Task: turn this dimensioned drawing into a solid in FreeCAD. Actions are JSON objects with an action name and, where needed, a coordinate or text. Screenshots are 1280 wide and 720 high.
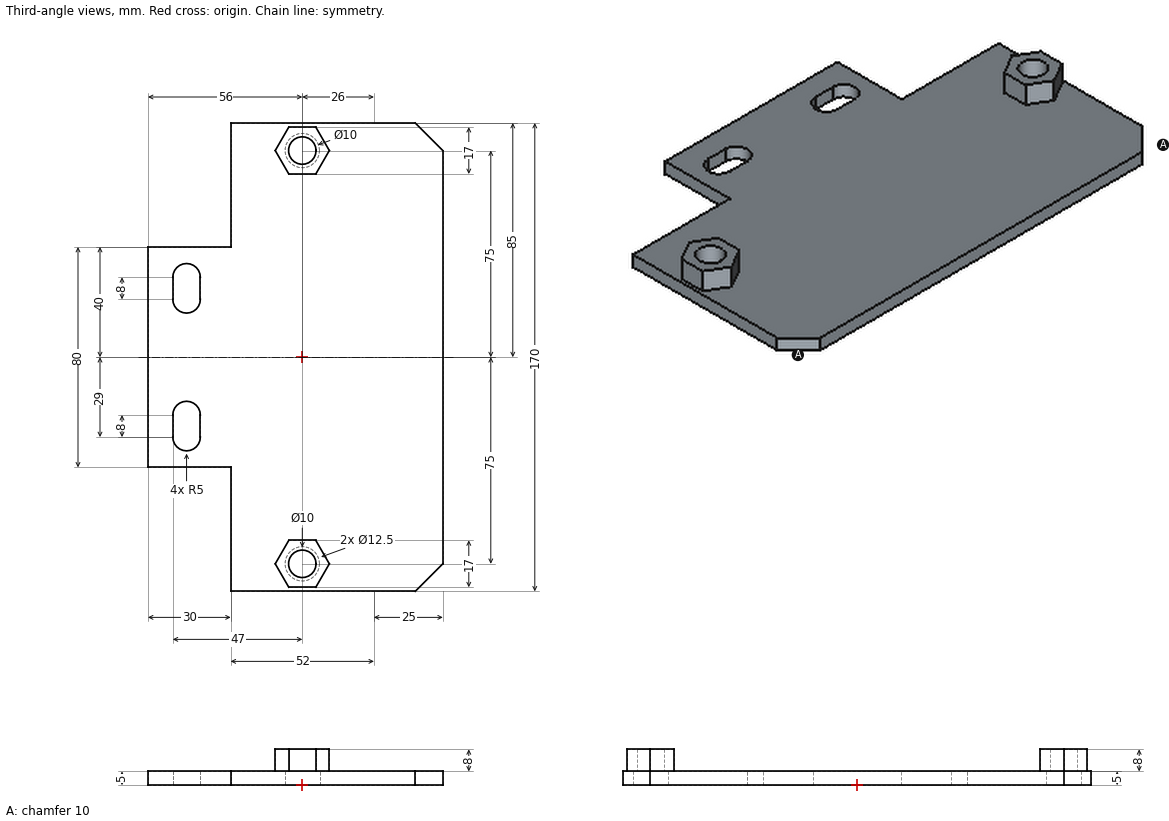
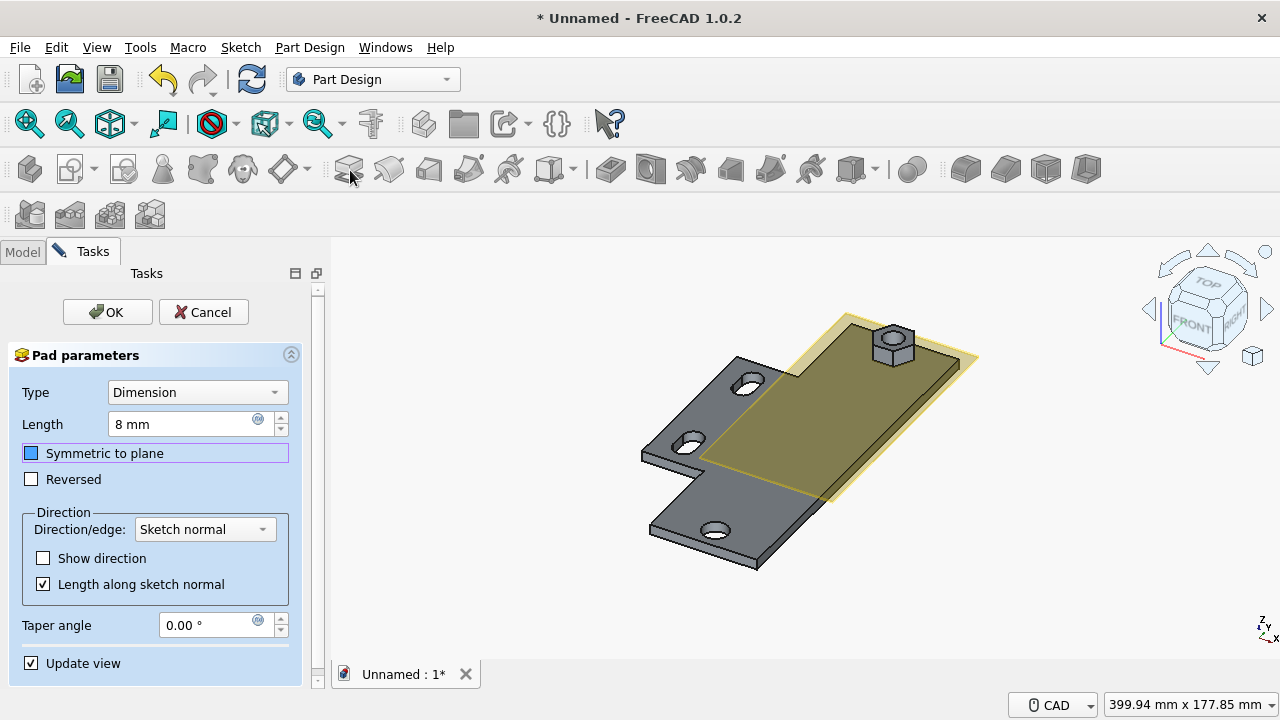
{"action": "left_click", "coordinate": [108, 312]}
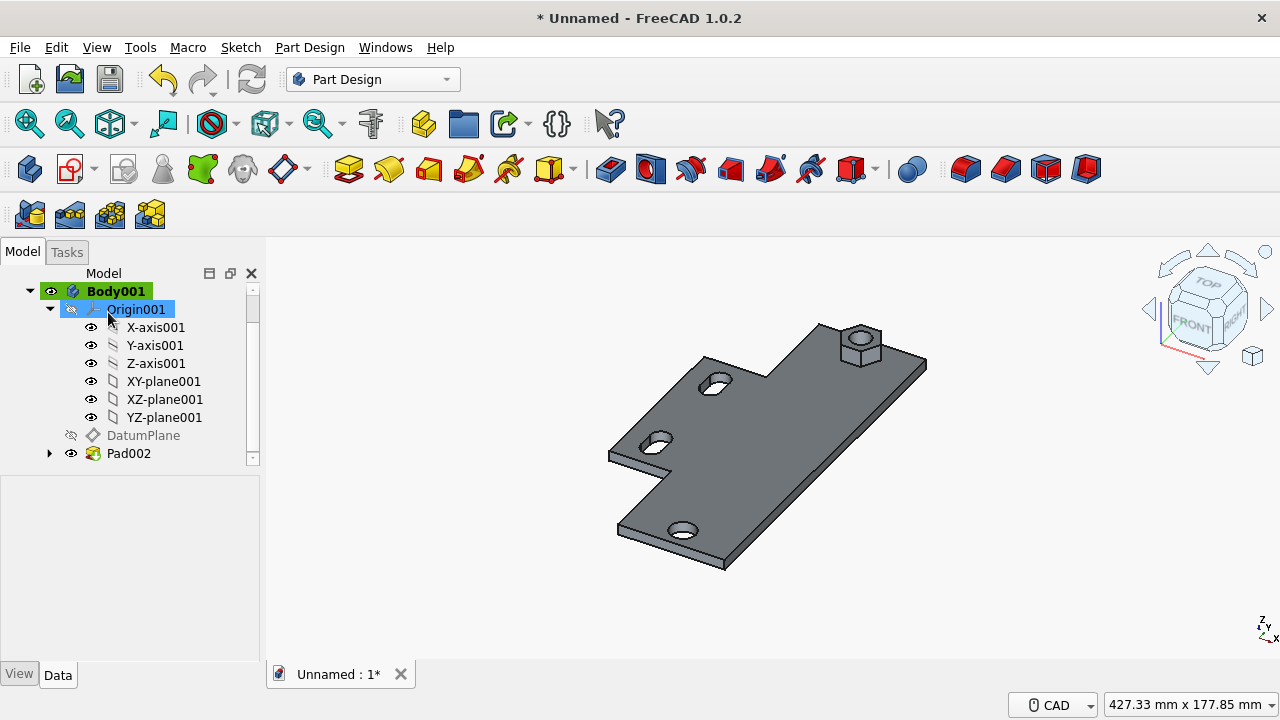
{"action": "left_click", "coordinate": [30, 124]}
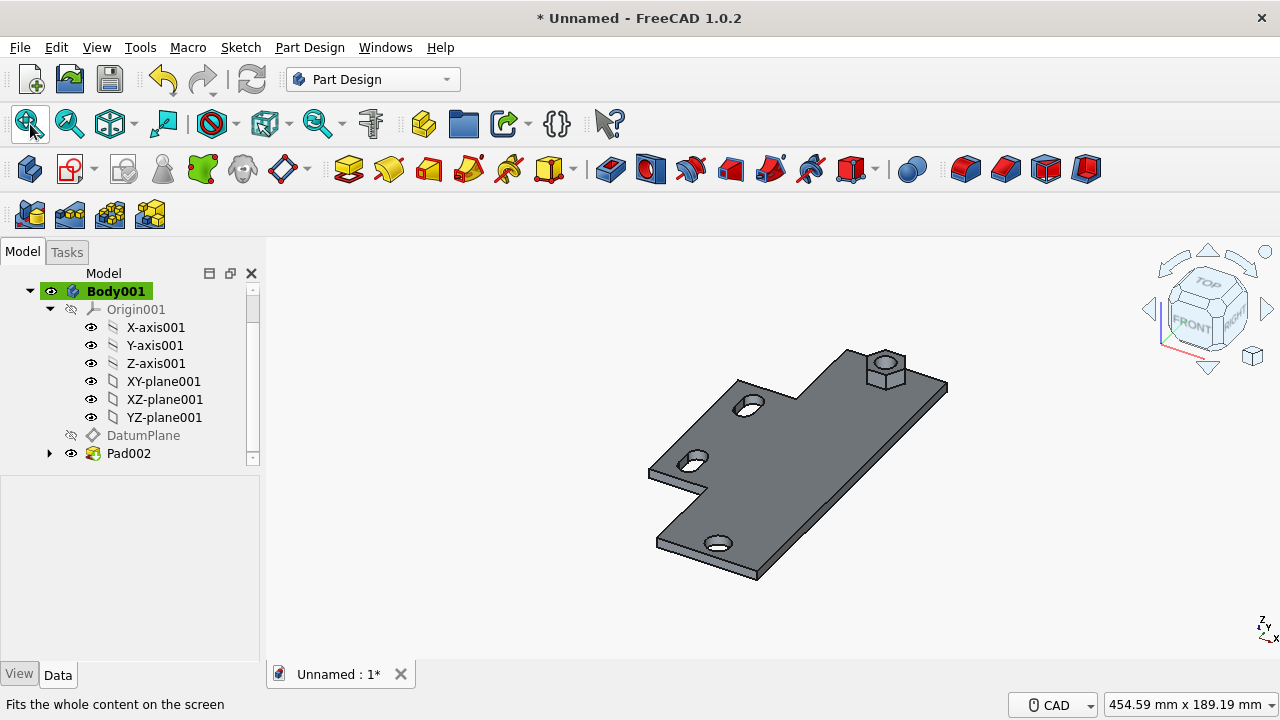
{"action": "left_click", "coordinate": [30, 170]}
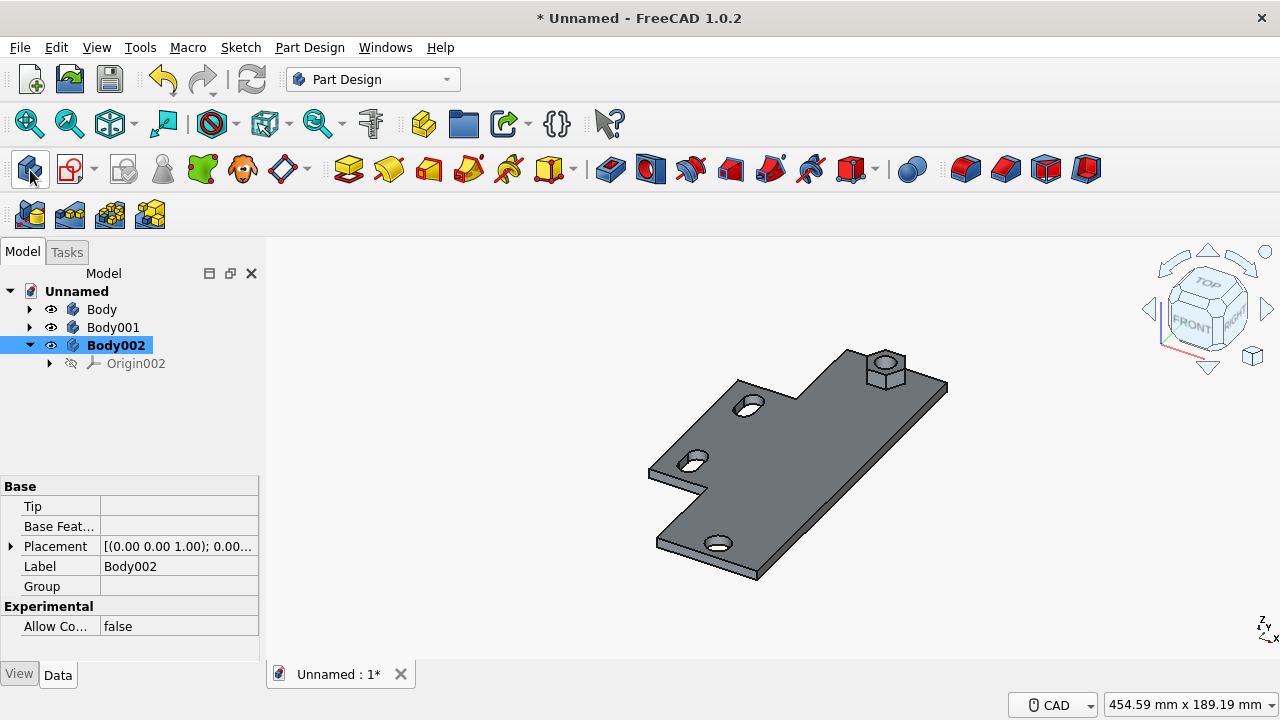
{"action": "left_click", "coordinate": [50, 363]}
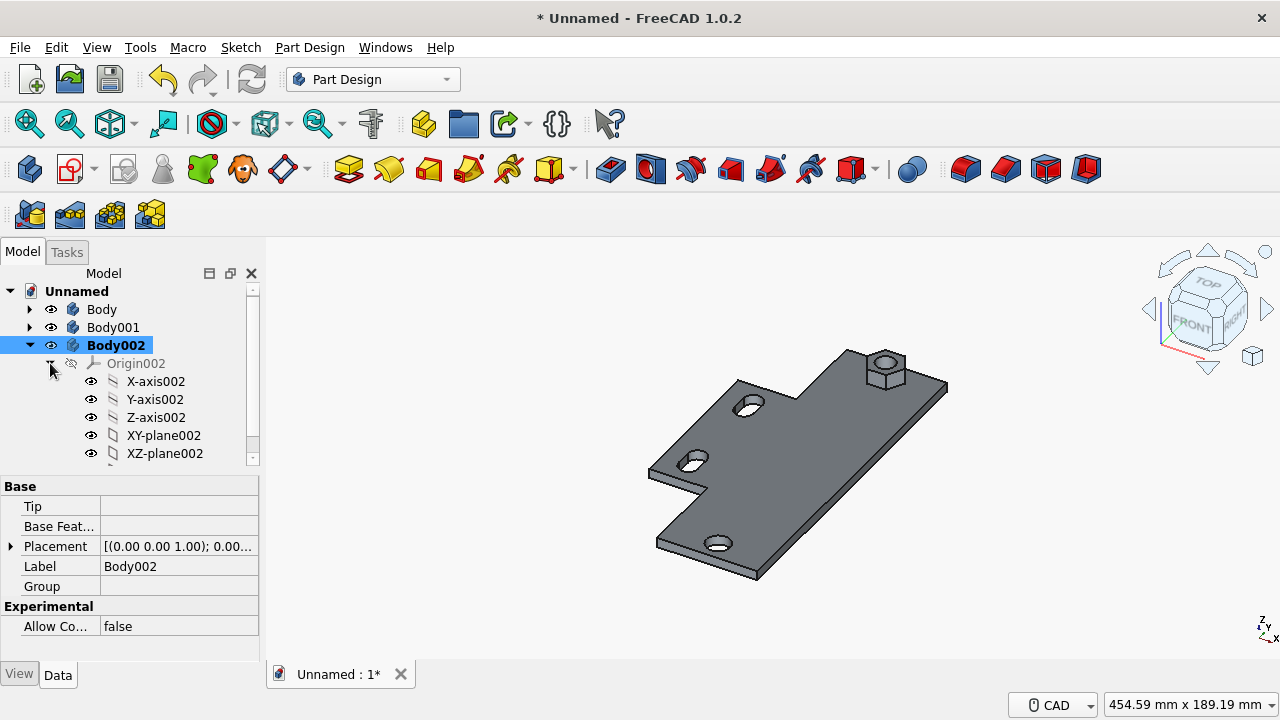
{"action": "left_click", "coordinate": [136, 435]}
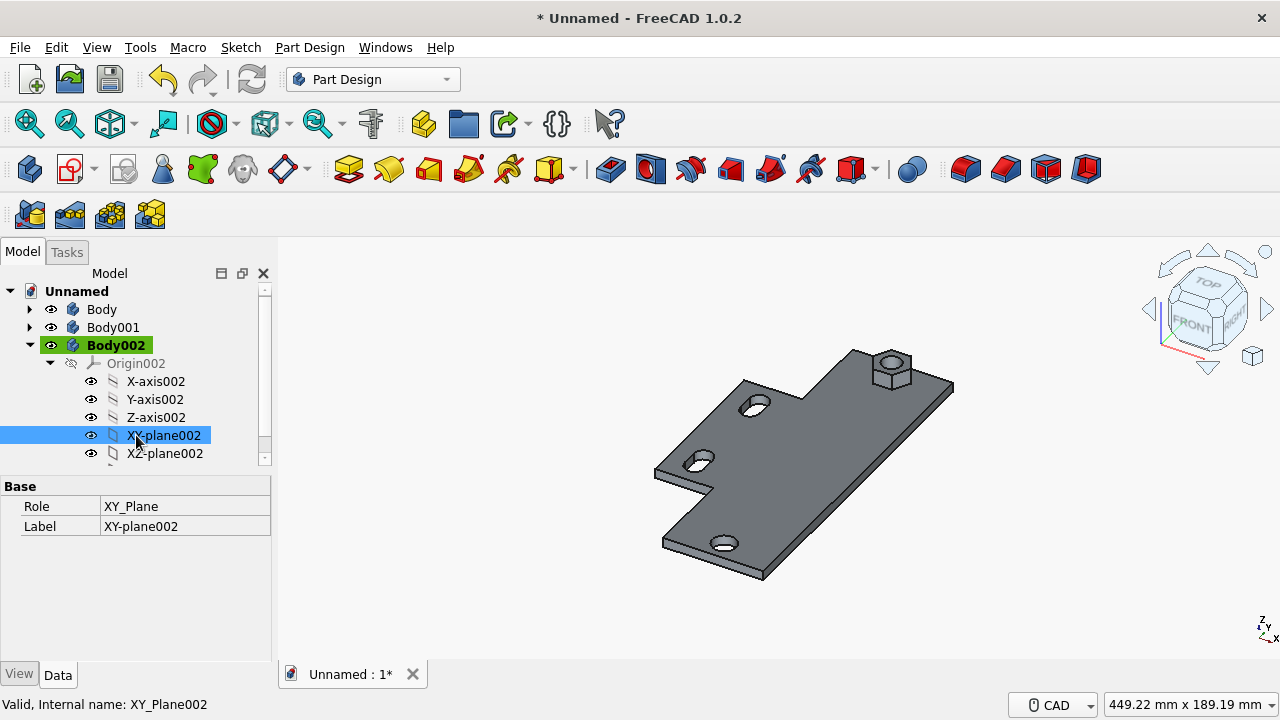
{"action": "left_click", "coordinate": [284, 170]}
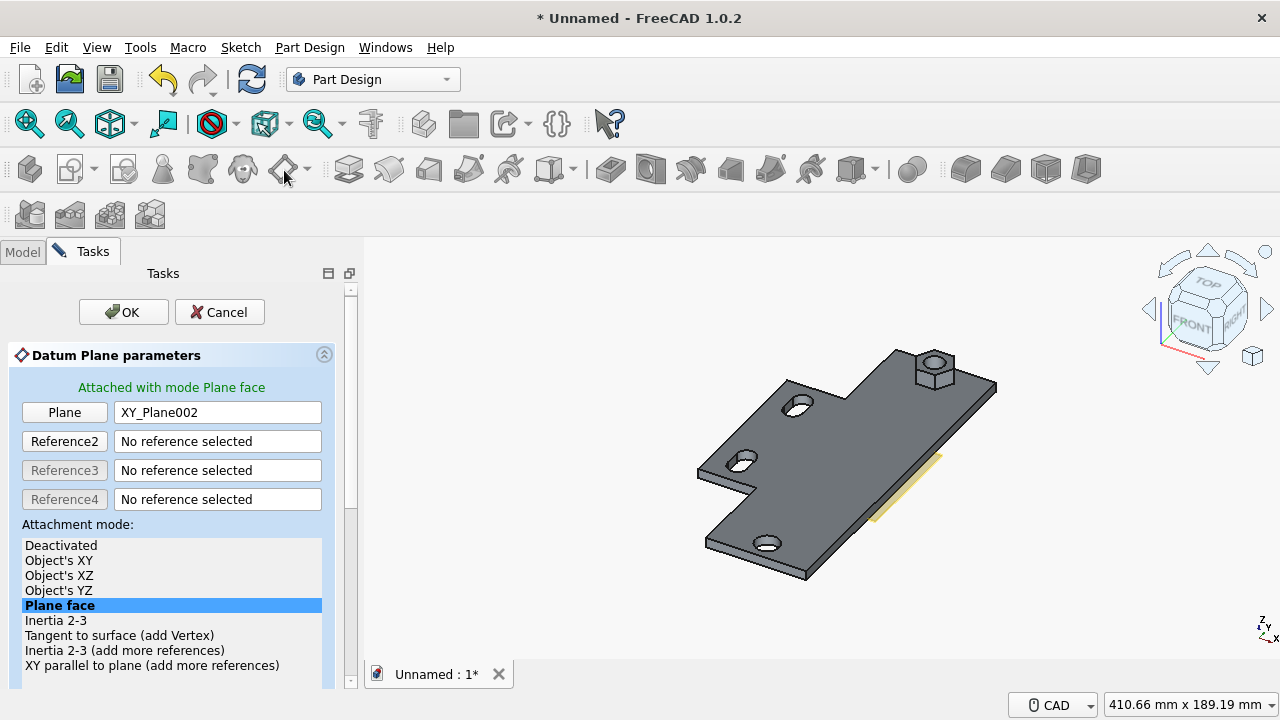
{"action": "scroll", "coordinate": [351, 486], "scroll_direction": "down", "scroll_amount": 4}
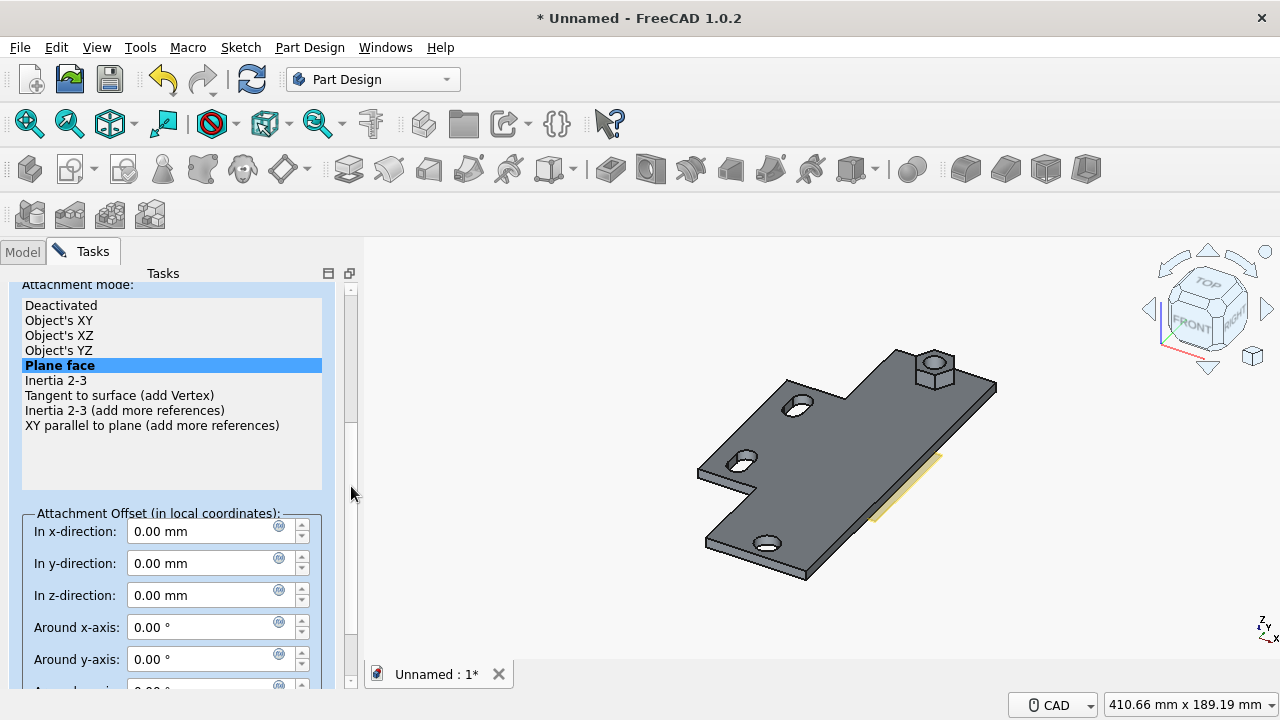
{"action": "triple_click", "coordinate": [210, 595]}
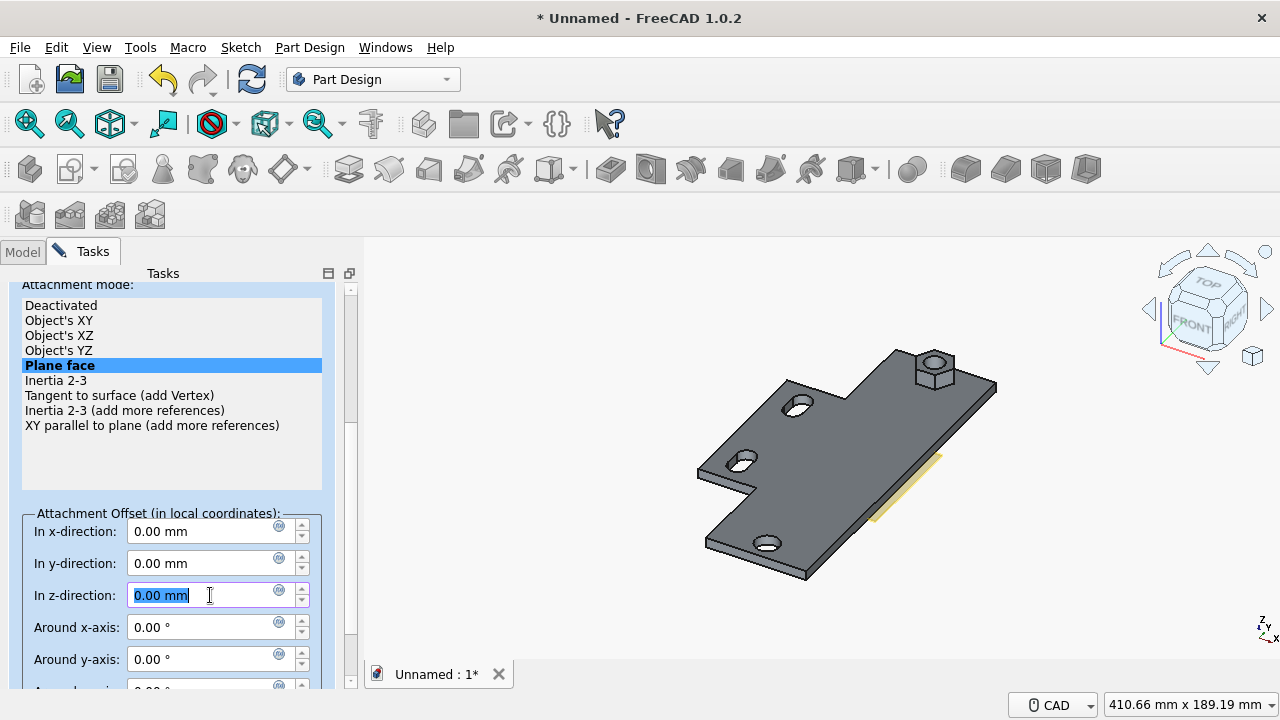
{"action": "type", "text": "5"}
{"action": "key", "text": "Tab"}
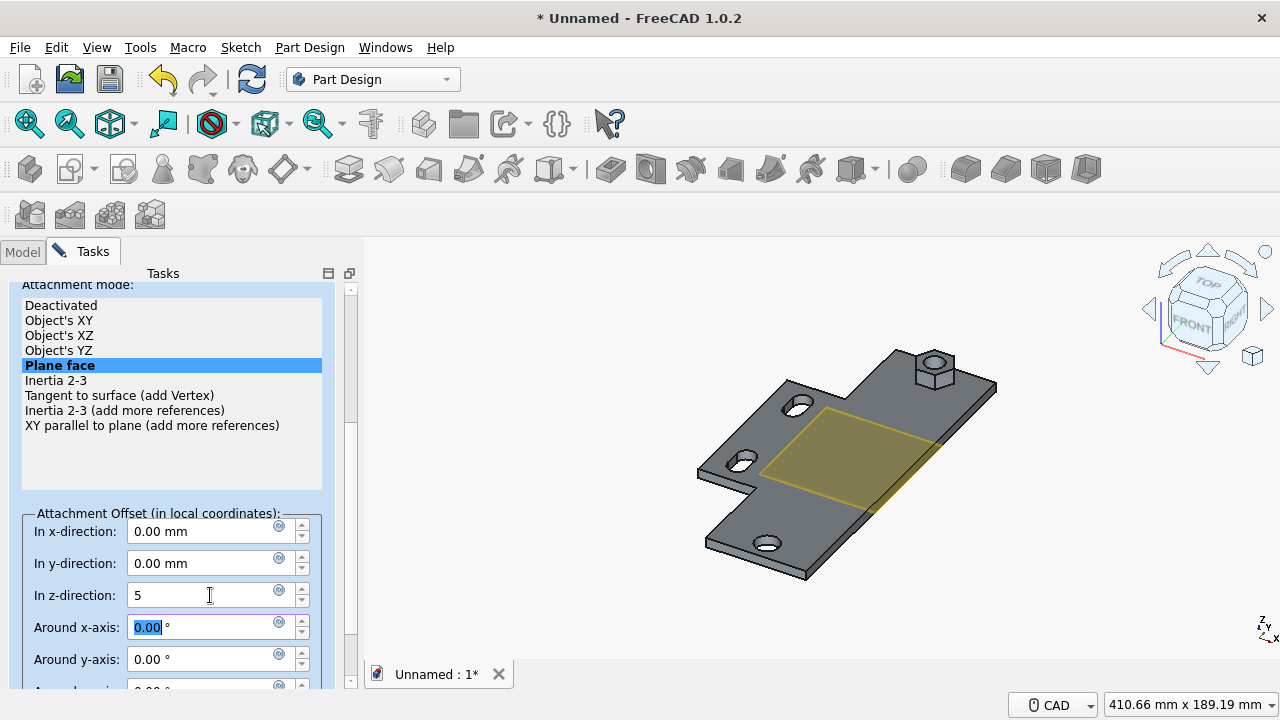
{"action": "scroll", "coordinate": [351, 486], "scroll_direction": "up", "scroll_amount": 5}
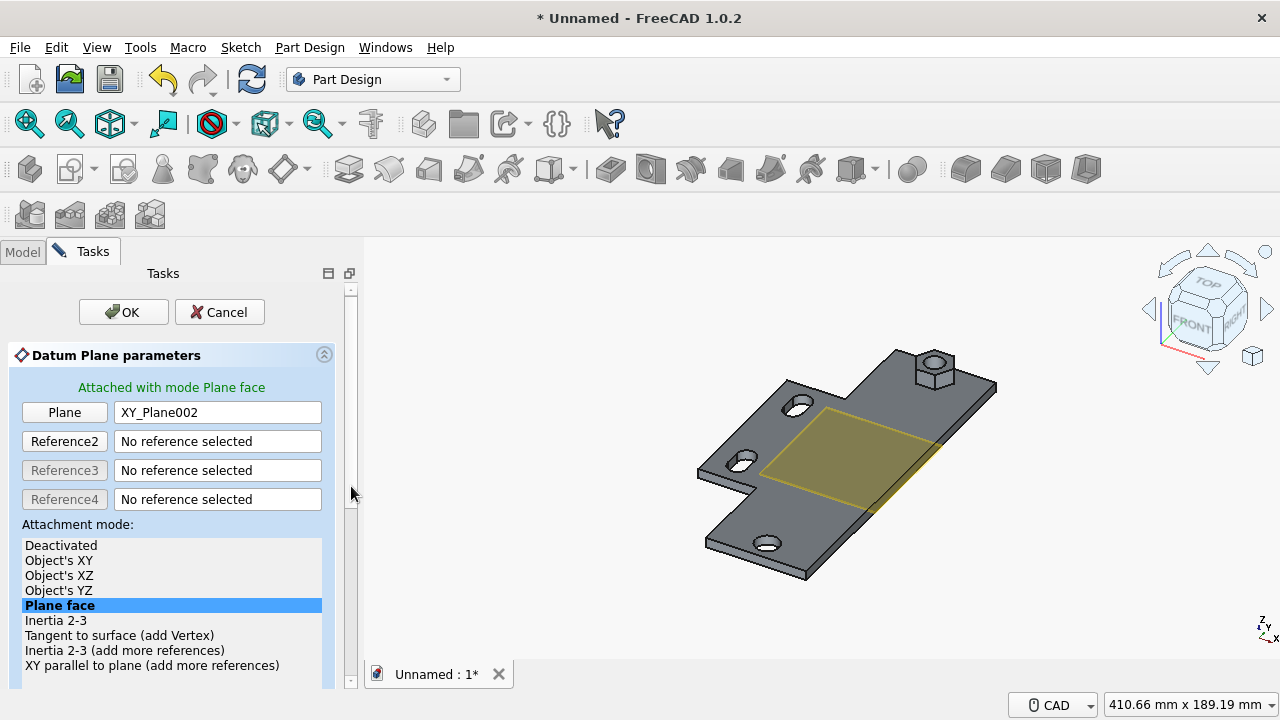
{"action": "left_click", "coordinate": [124, 312]}